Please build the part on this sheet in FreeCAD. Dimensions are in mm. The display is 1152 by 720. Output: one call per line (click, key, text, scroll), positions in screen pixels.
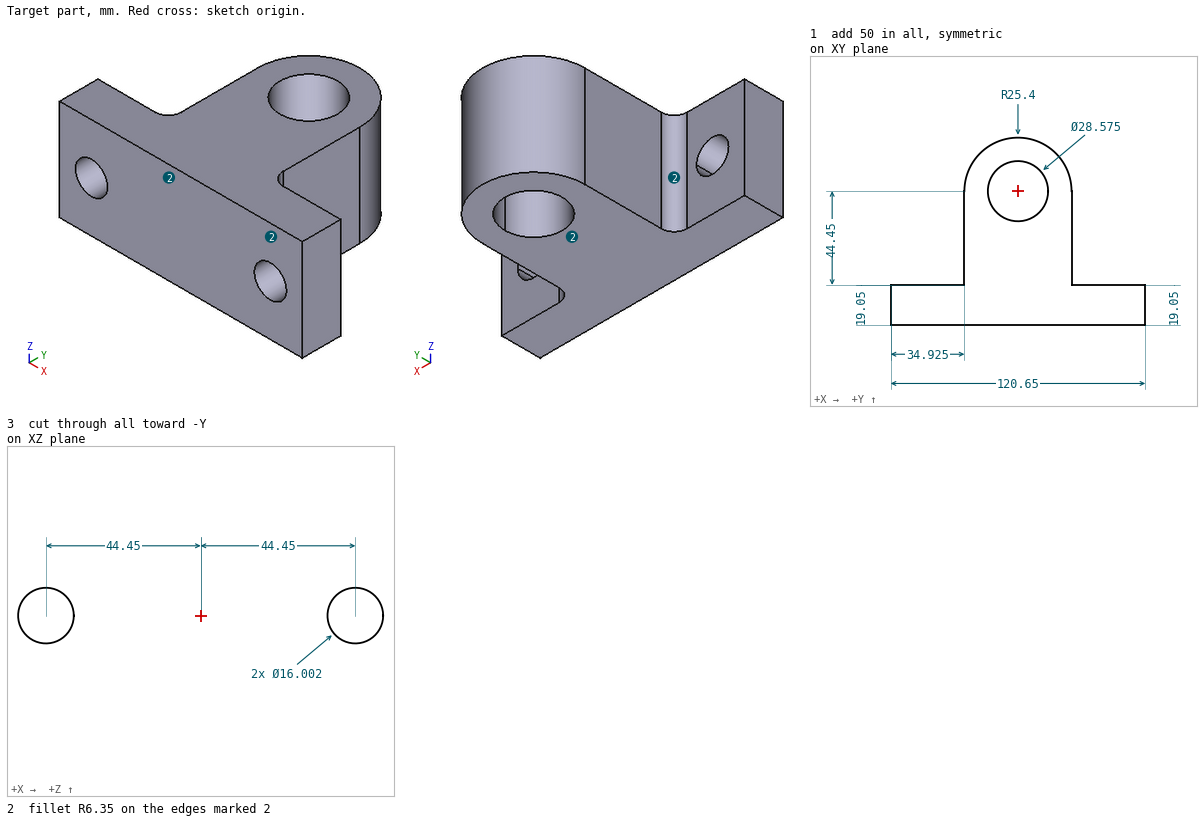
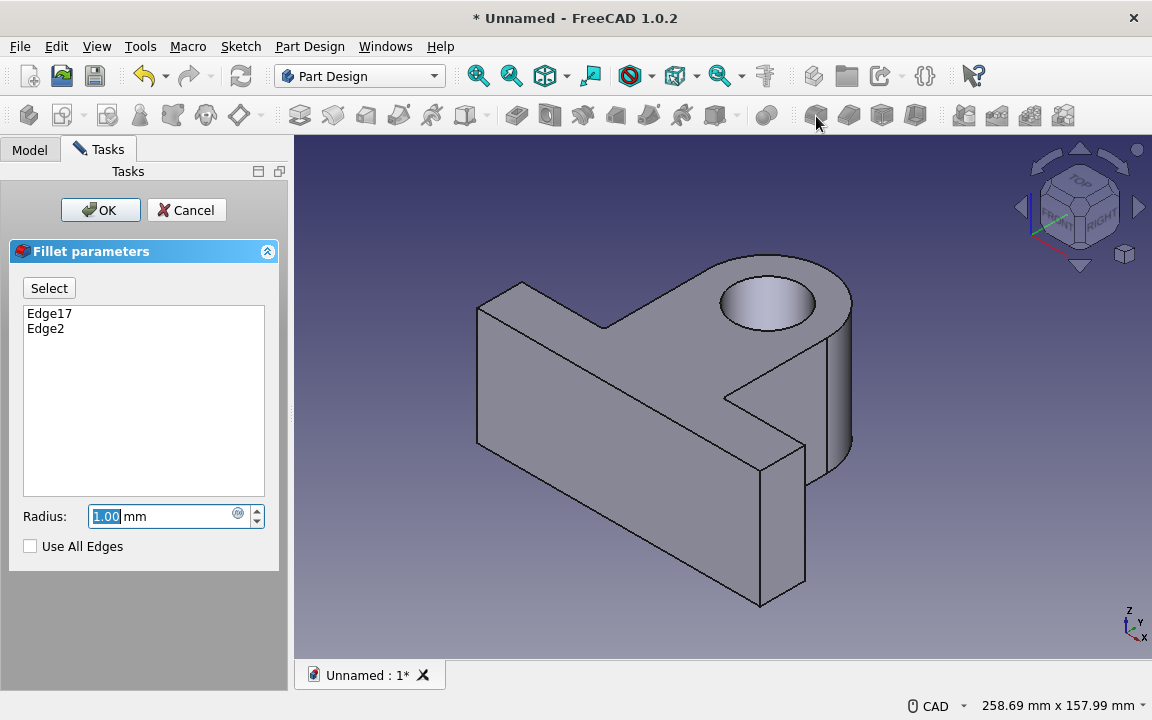
text(6.35)
key(Tab)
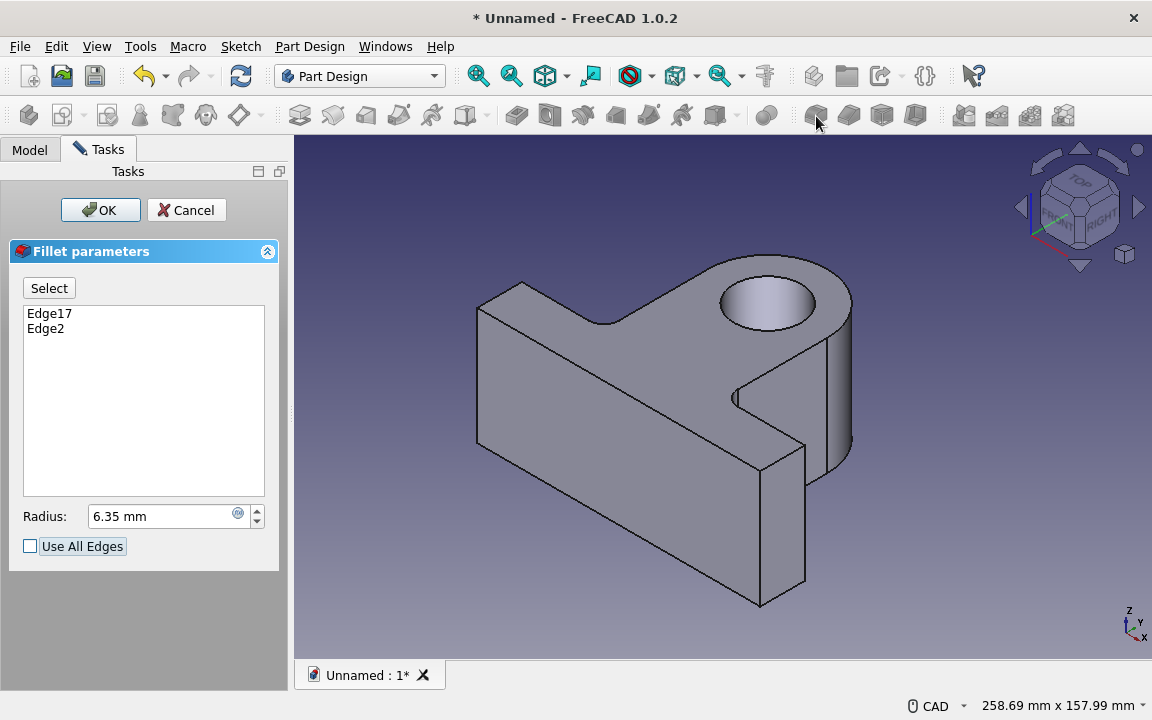
click(101, 210)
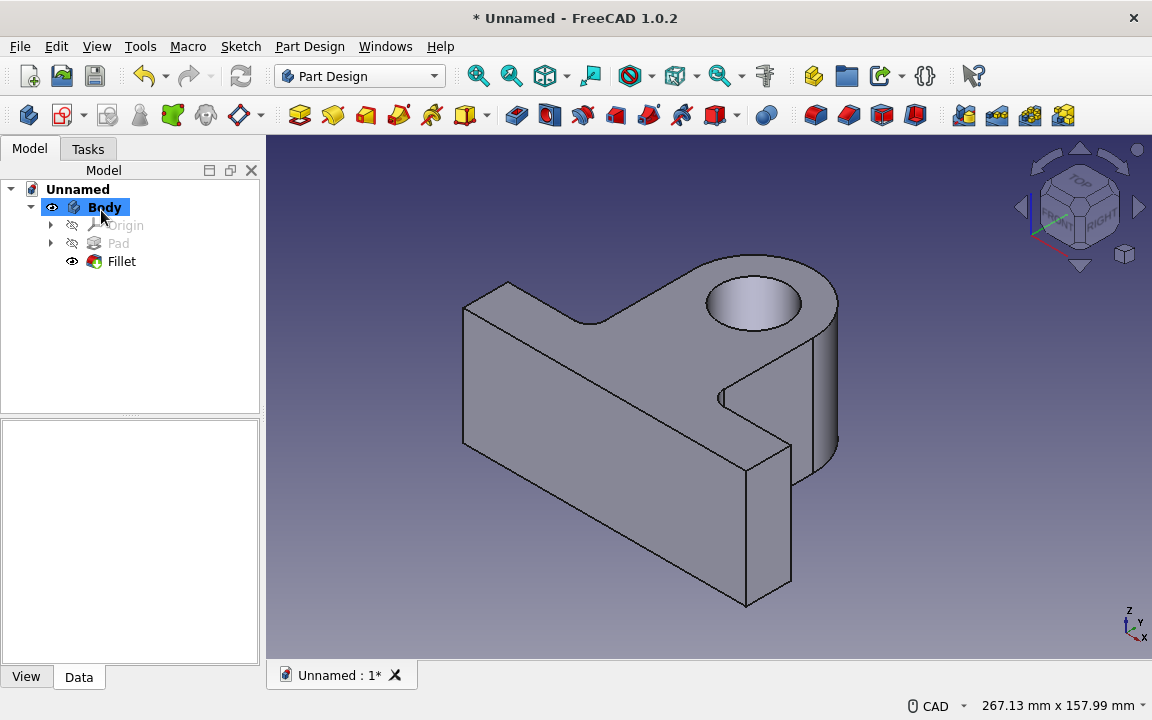
click(62, 116)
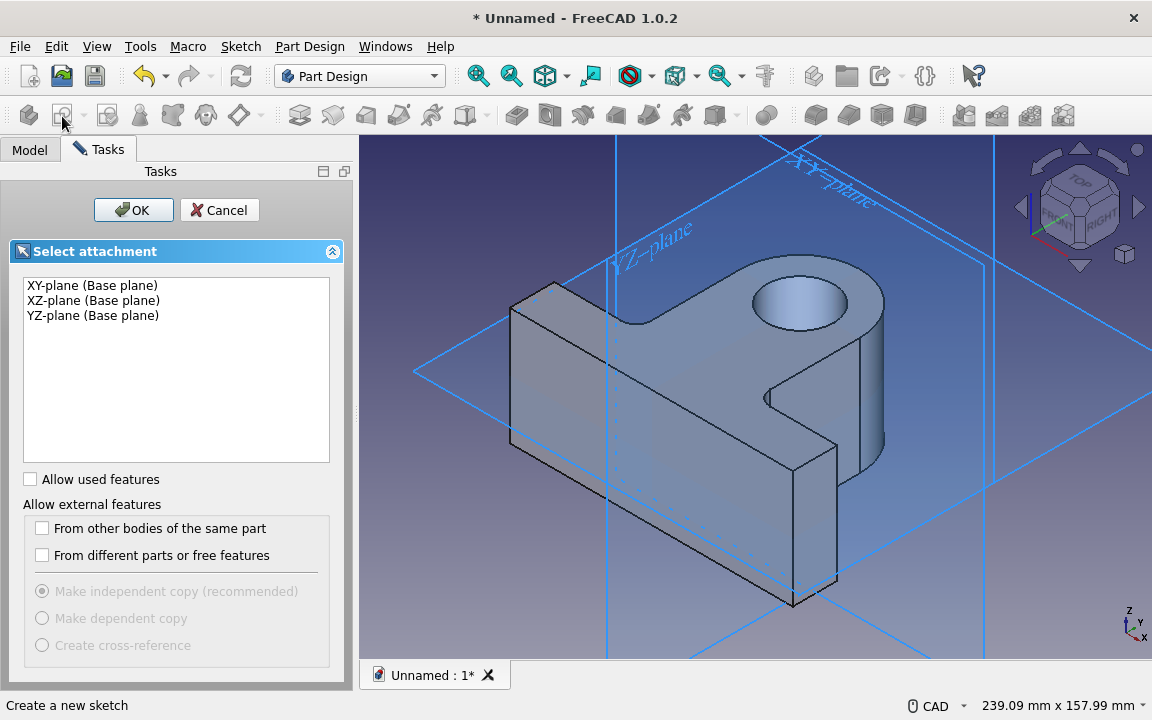
click(84, 300)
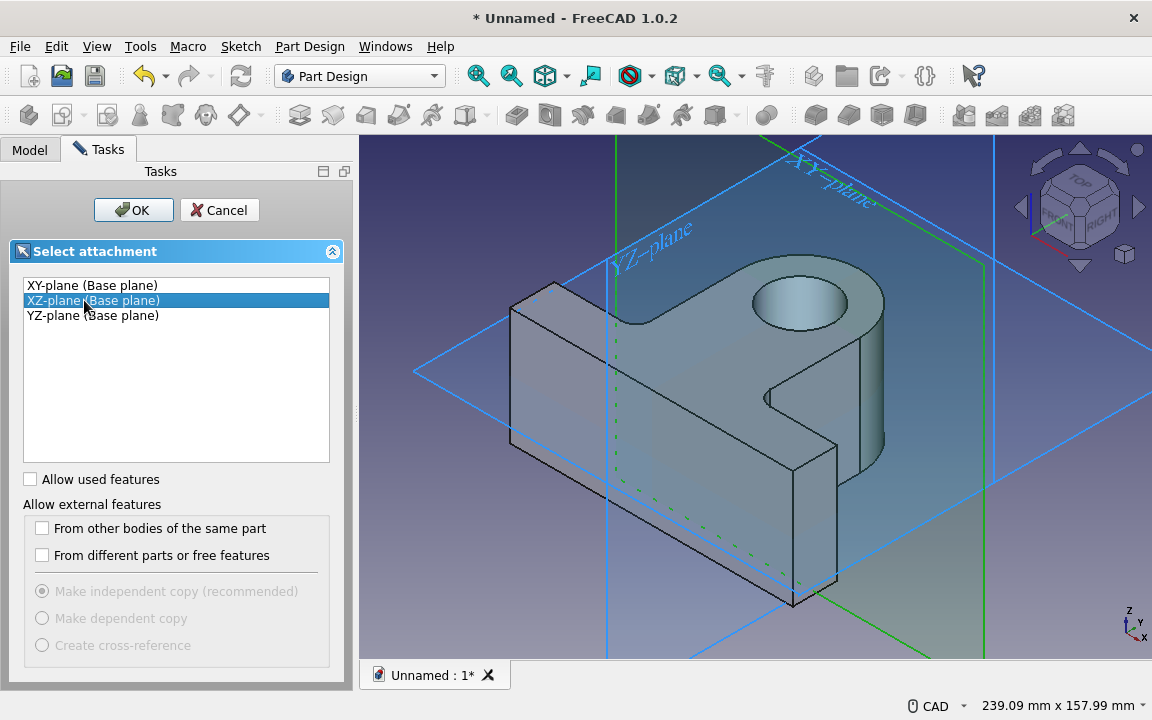
click(134, 210)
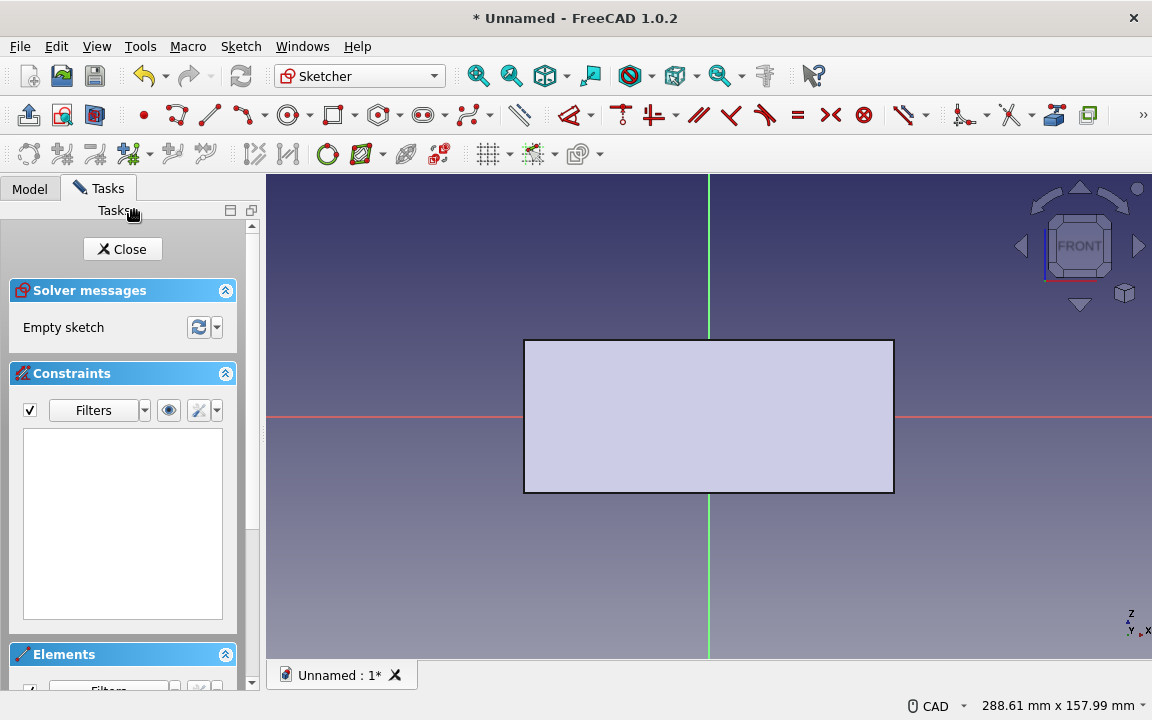
click(95, 116)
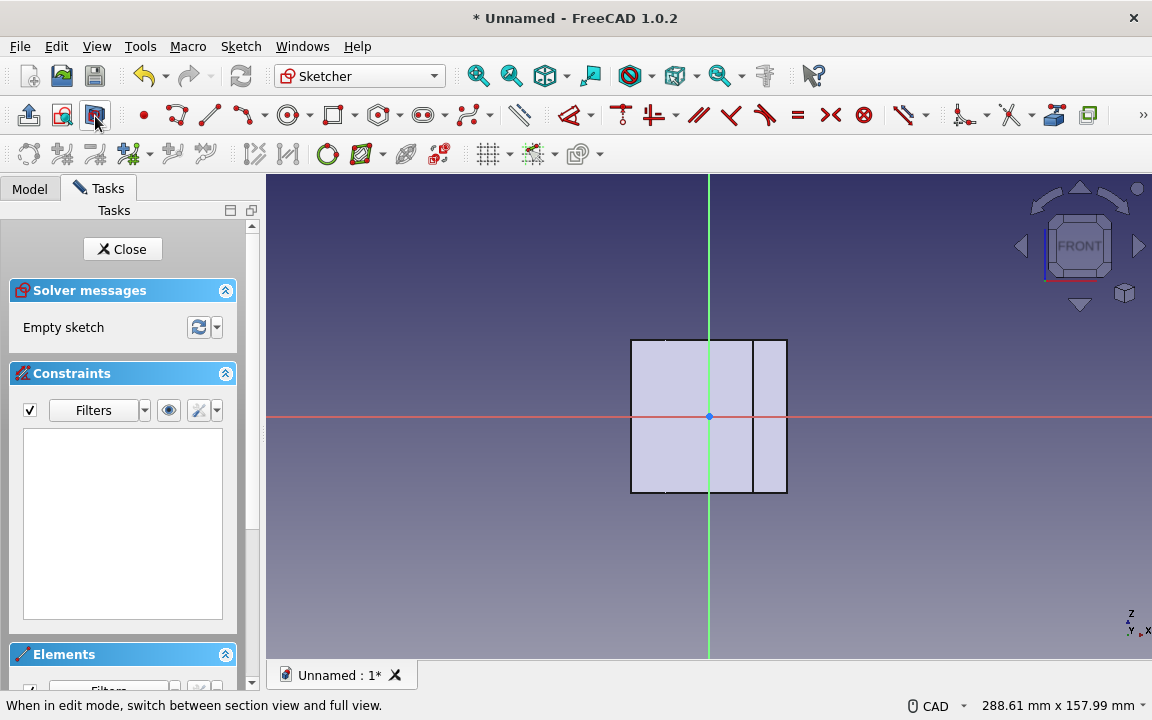
scroll(848, 416, up, 2)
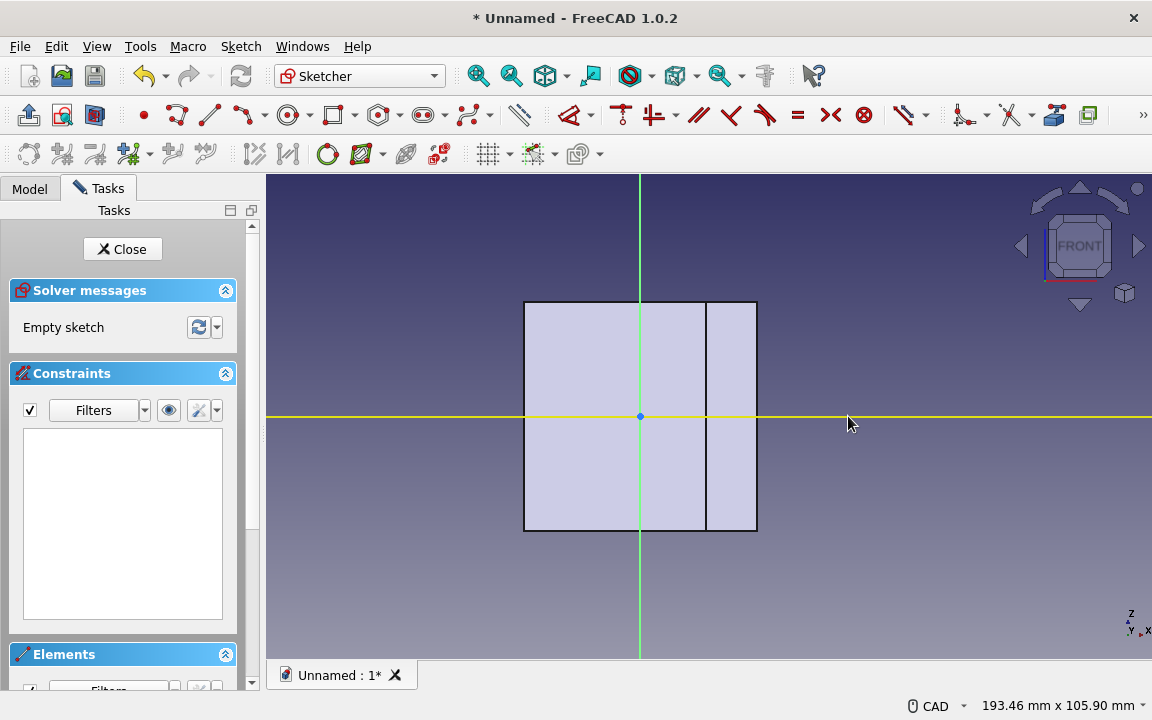
click(288, 116)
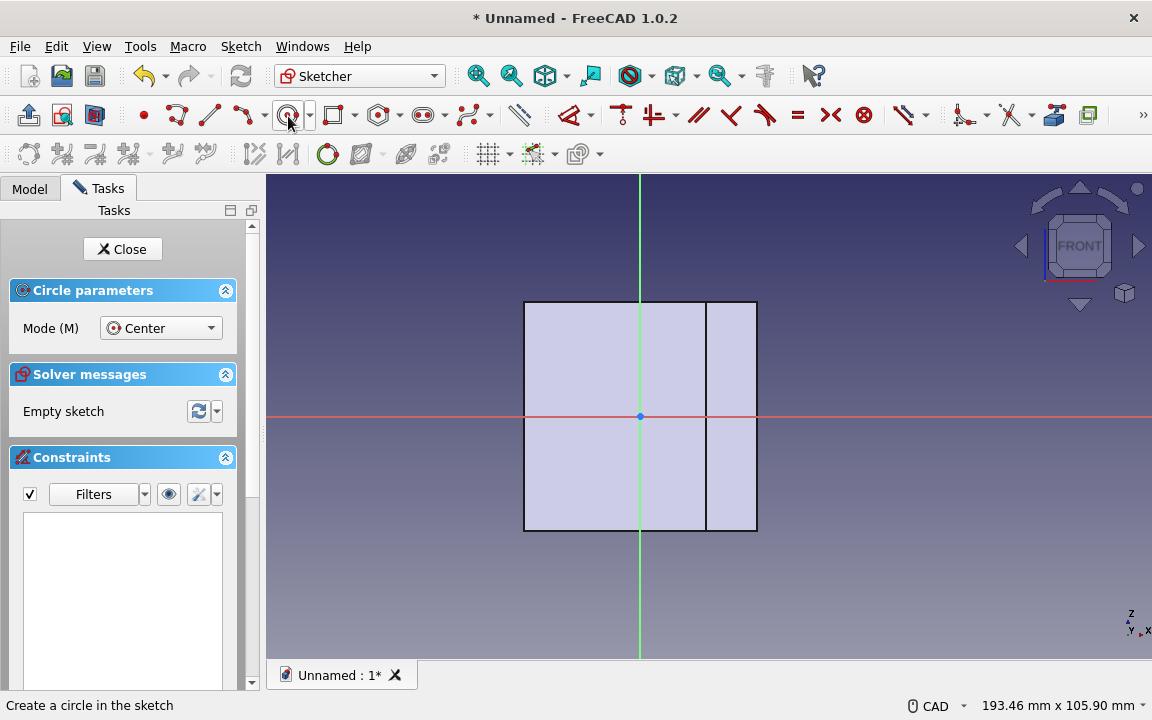
click(844, 416)
move(870, 391)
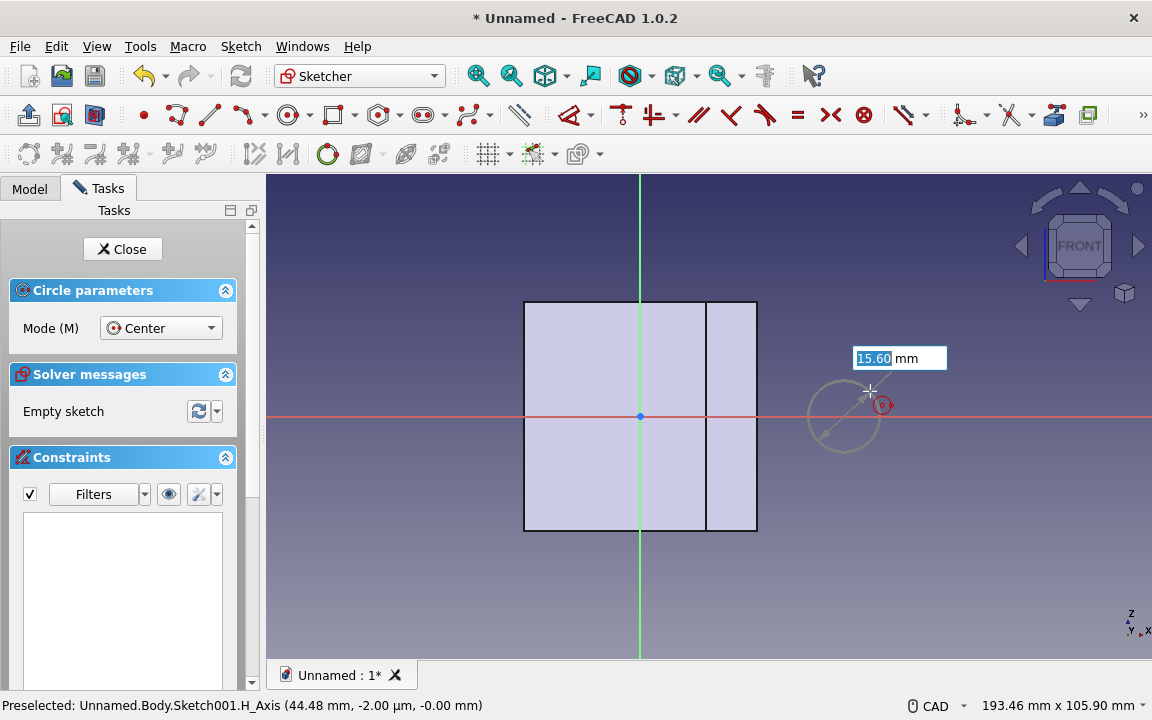
text(16.002)
key(Return)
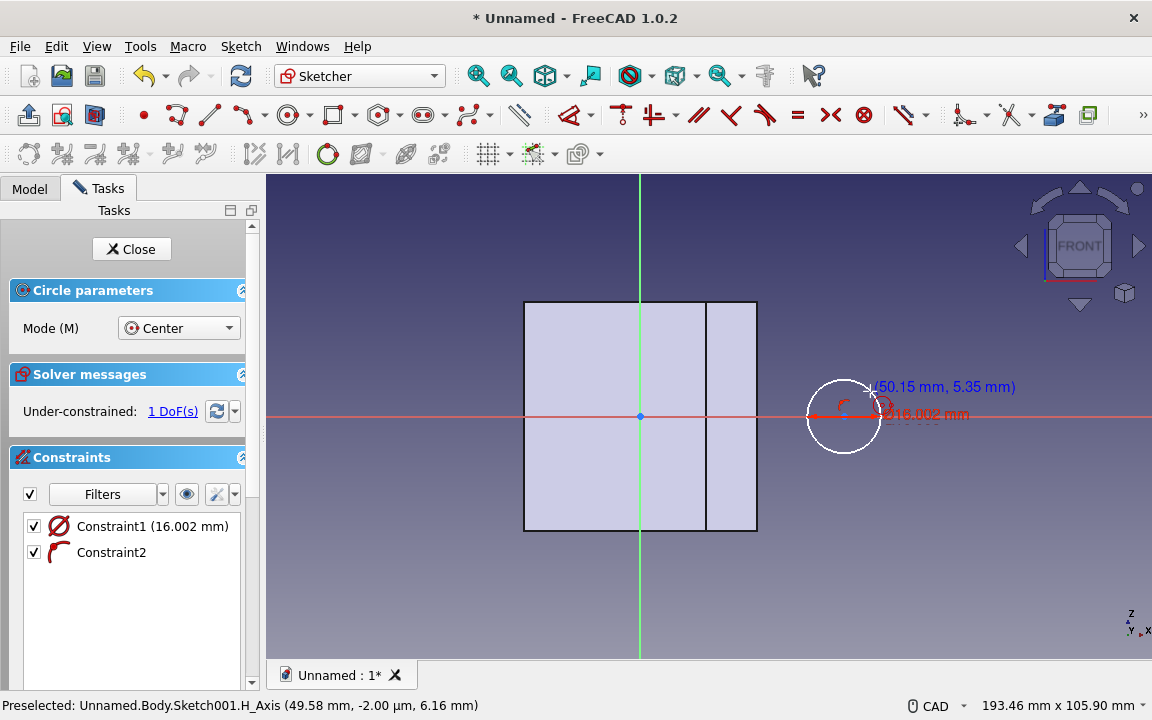
click(437, 416)
move(463, 391)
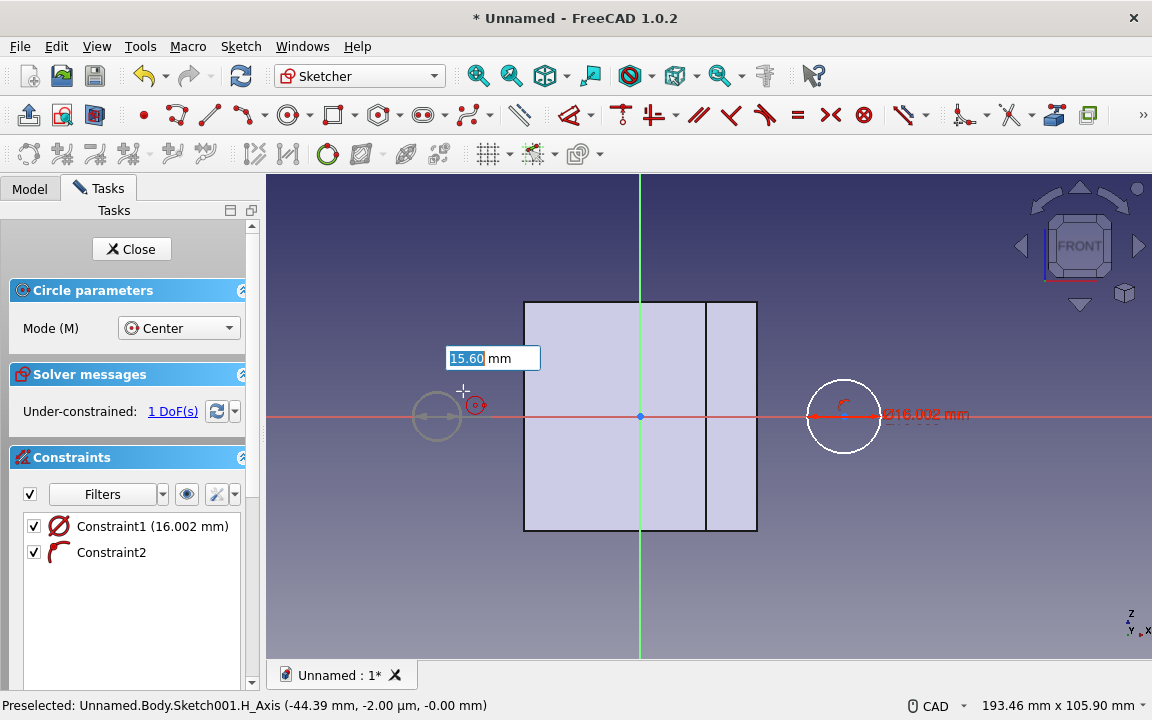
text(16.002)
key(Return)
key(Escape)